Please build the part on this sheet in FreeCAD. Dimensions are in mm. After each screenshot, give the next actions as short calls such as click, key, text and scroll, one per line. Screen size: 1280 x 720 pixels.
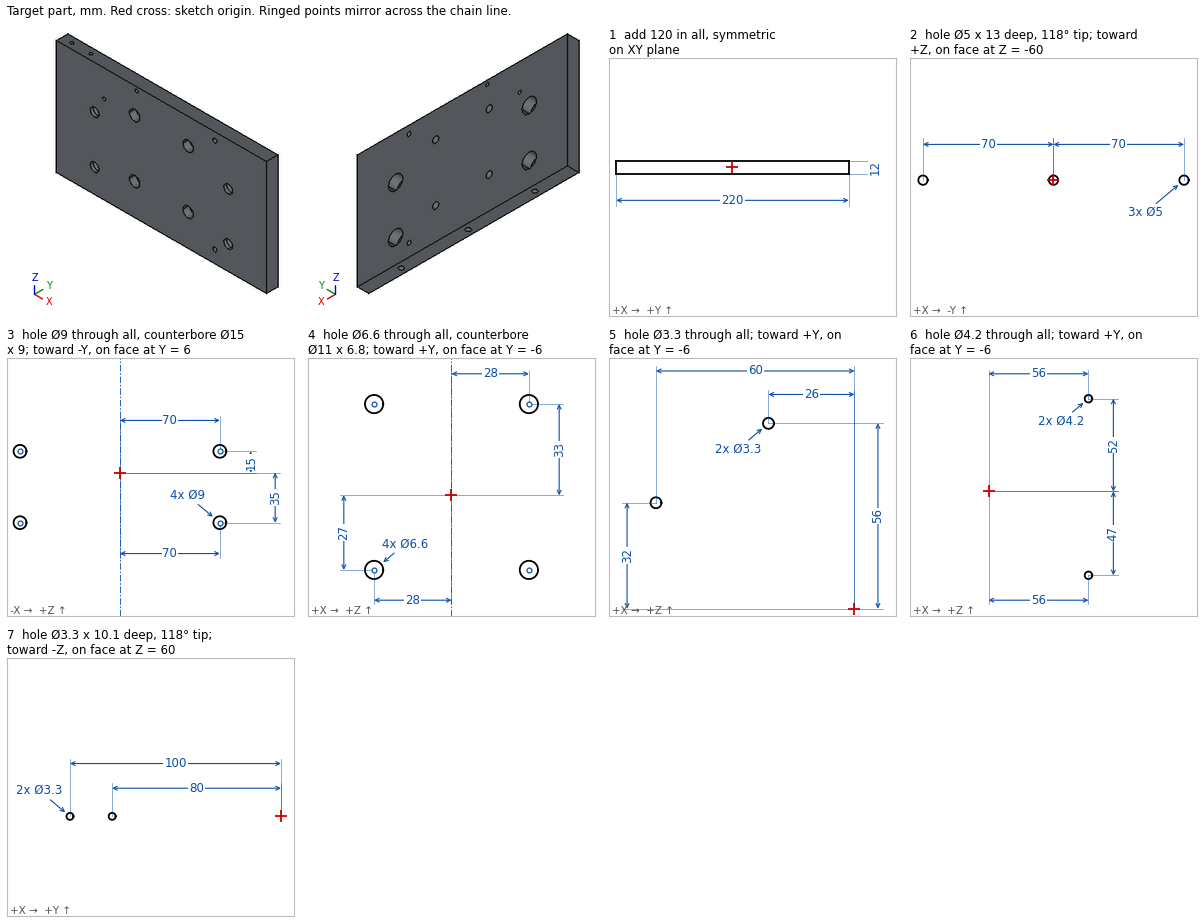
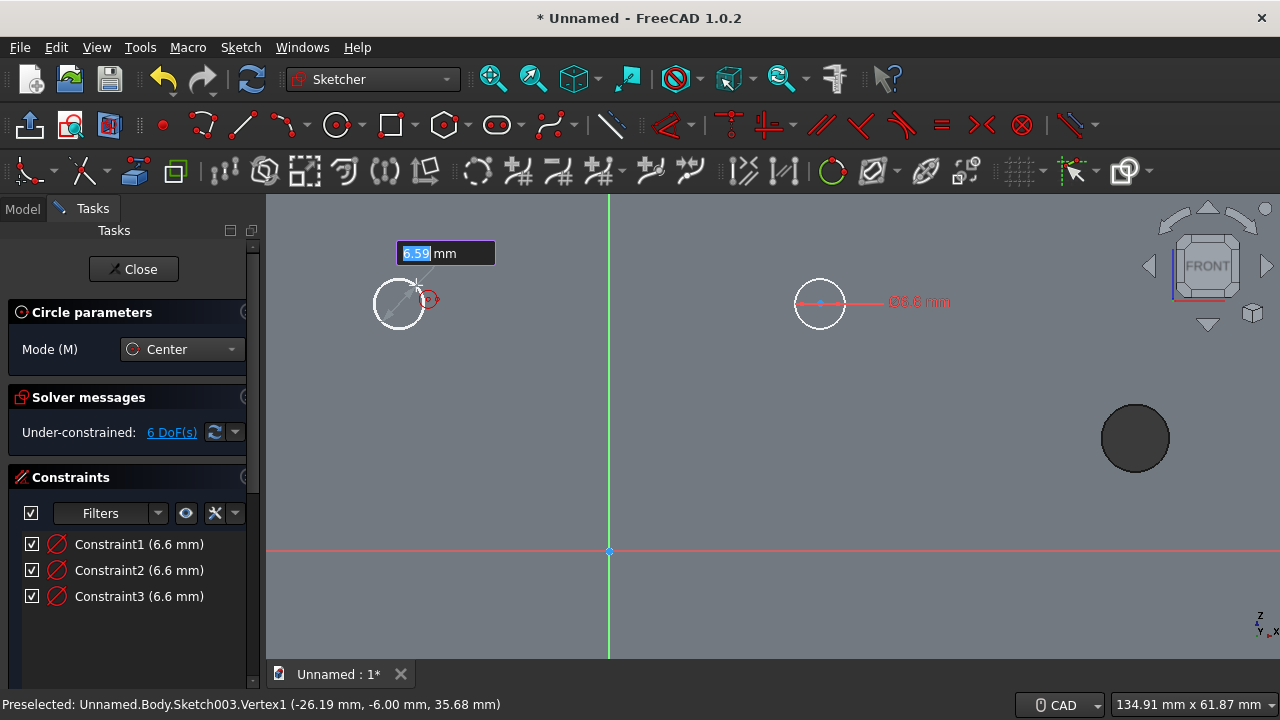
text(6.6)
key(Return)
key(Escape)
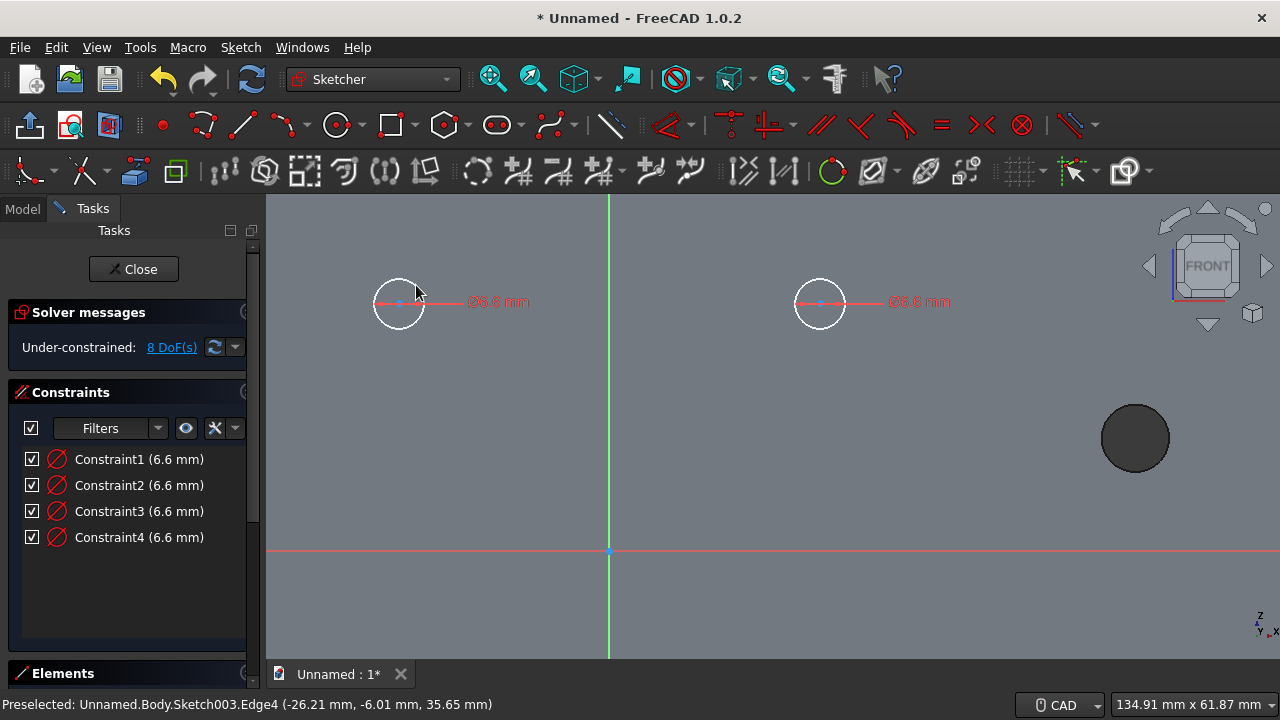
scroll(820, 302, down, 3)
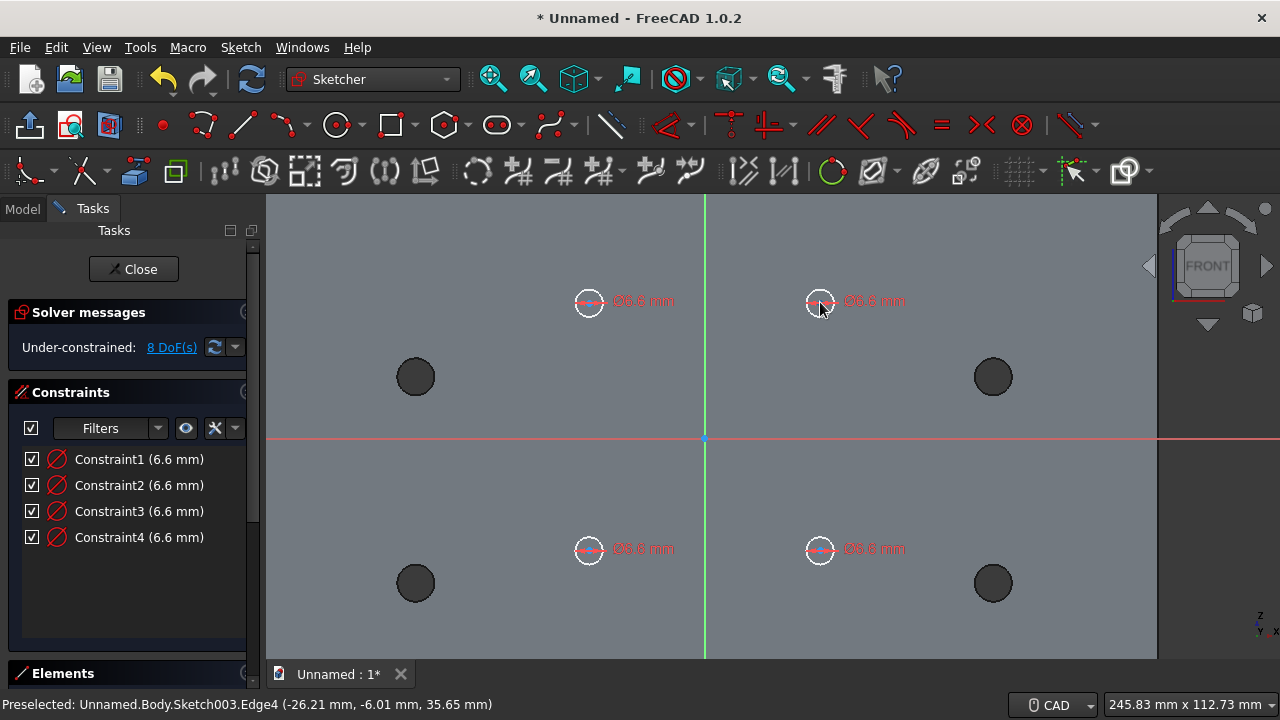
click(589, 551)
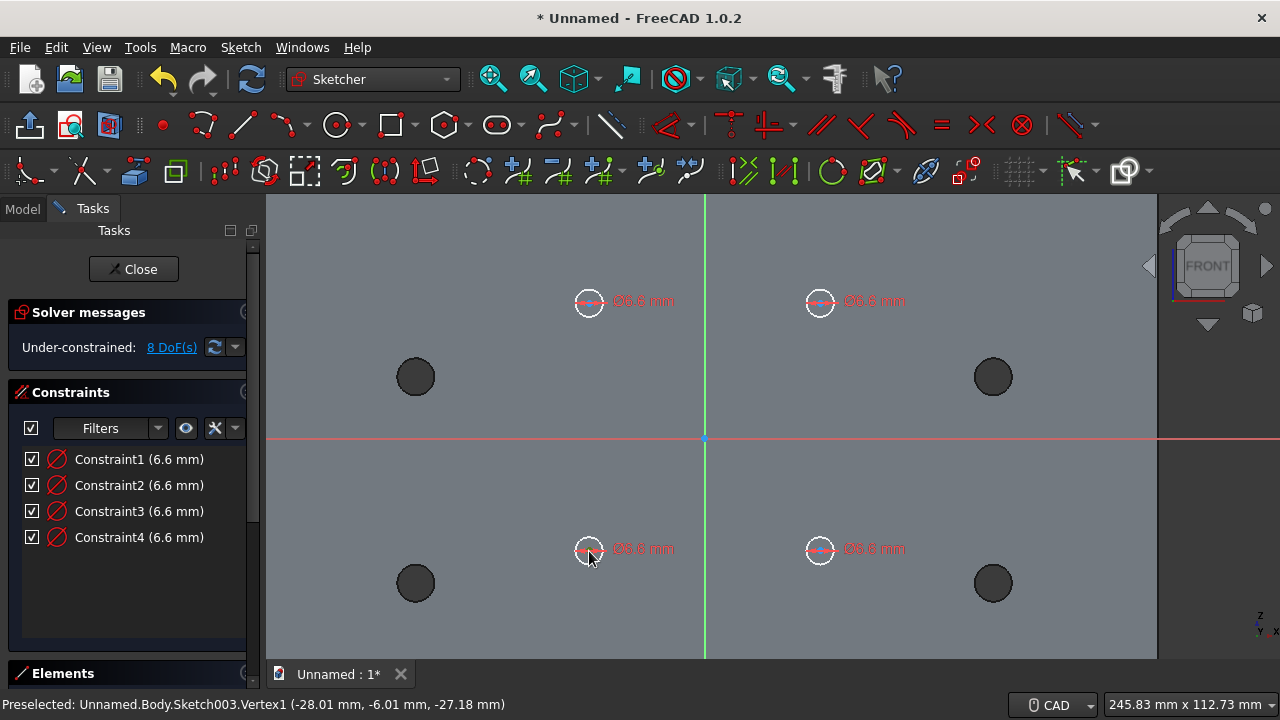
click(820, 551)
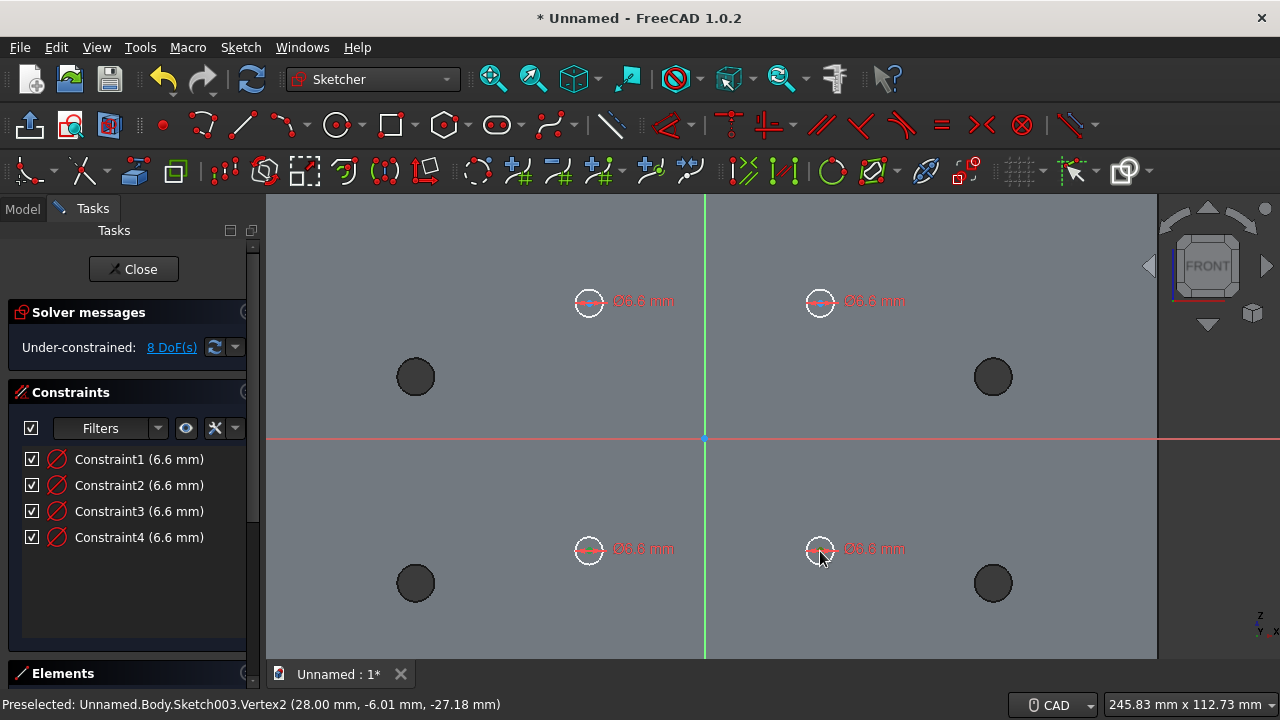
click(705, 602)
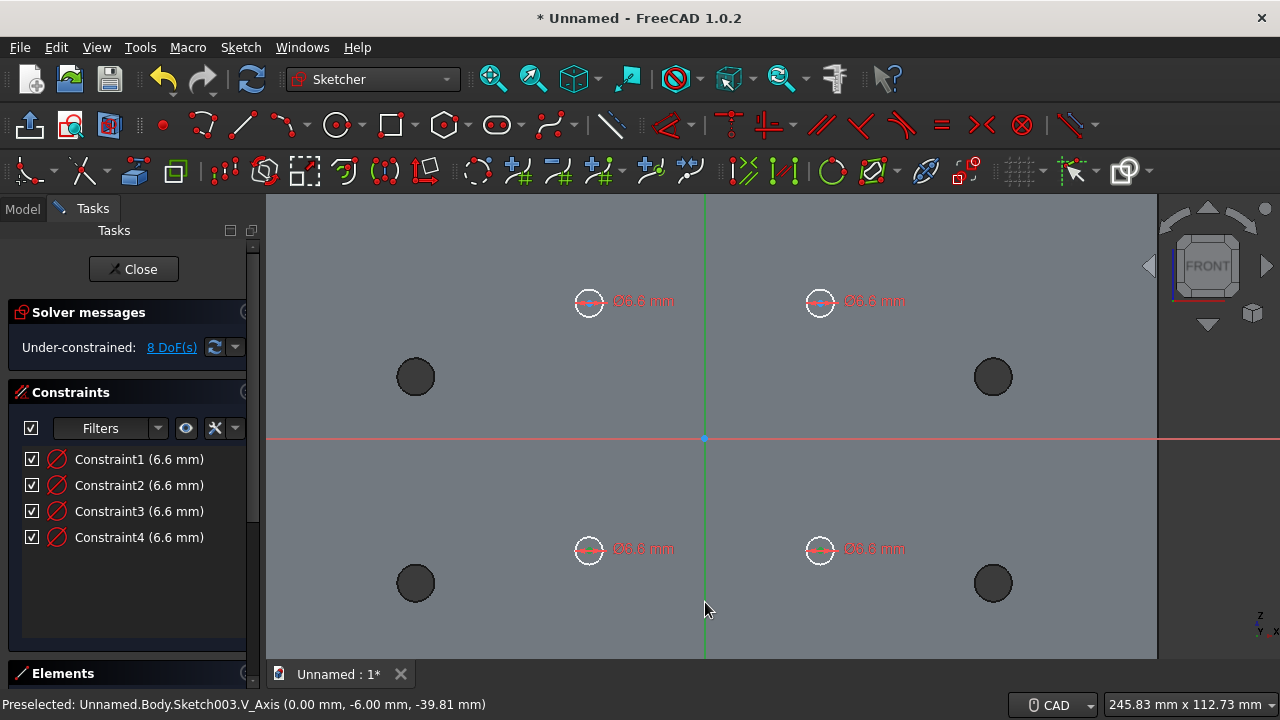
key(s)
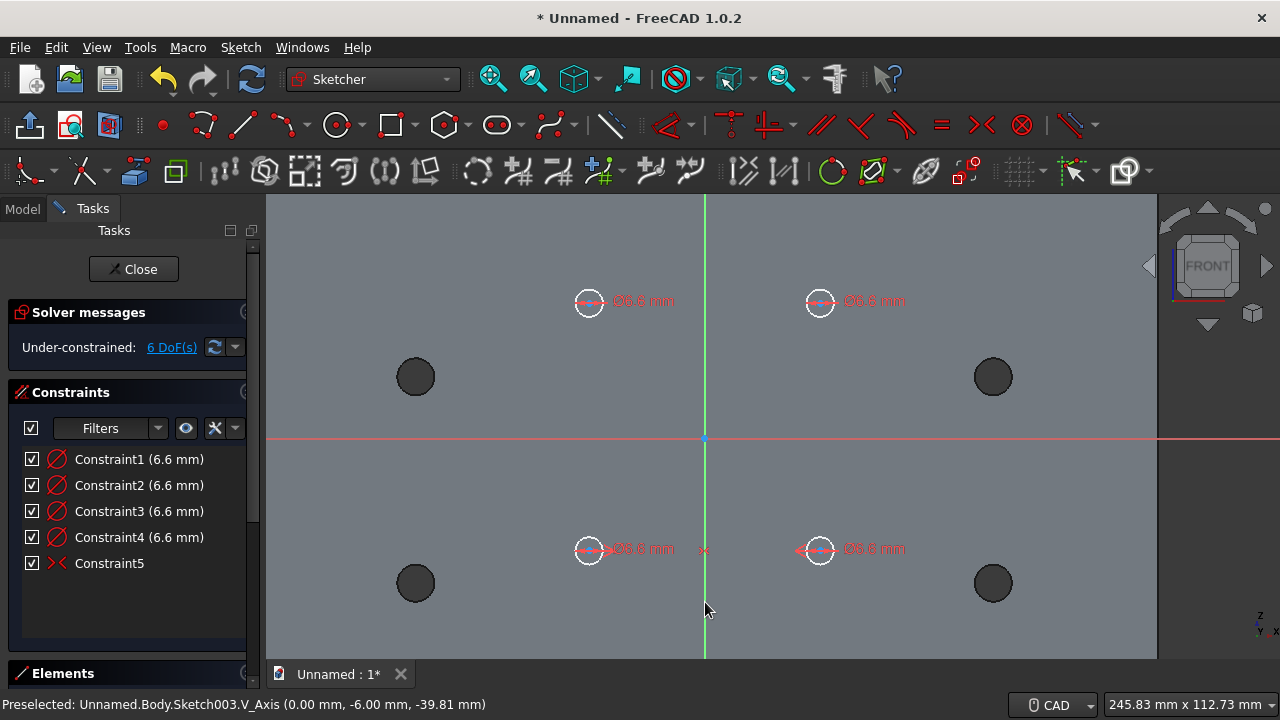
click(820, 303)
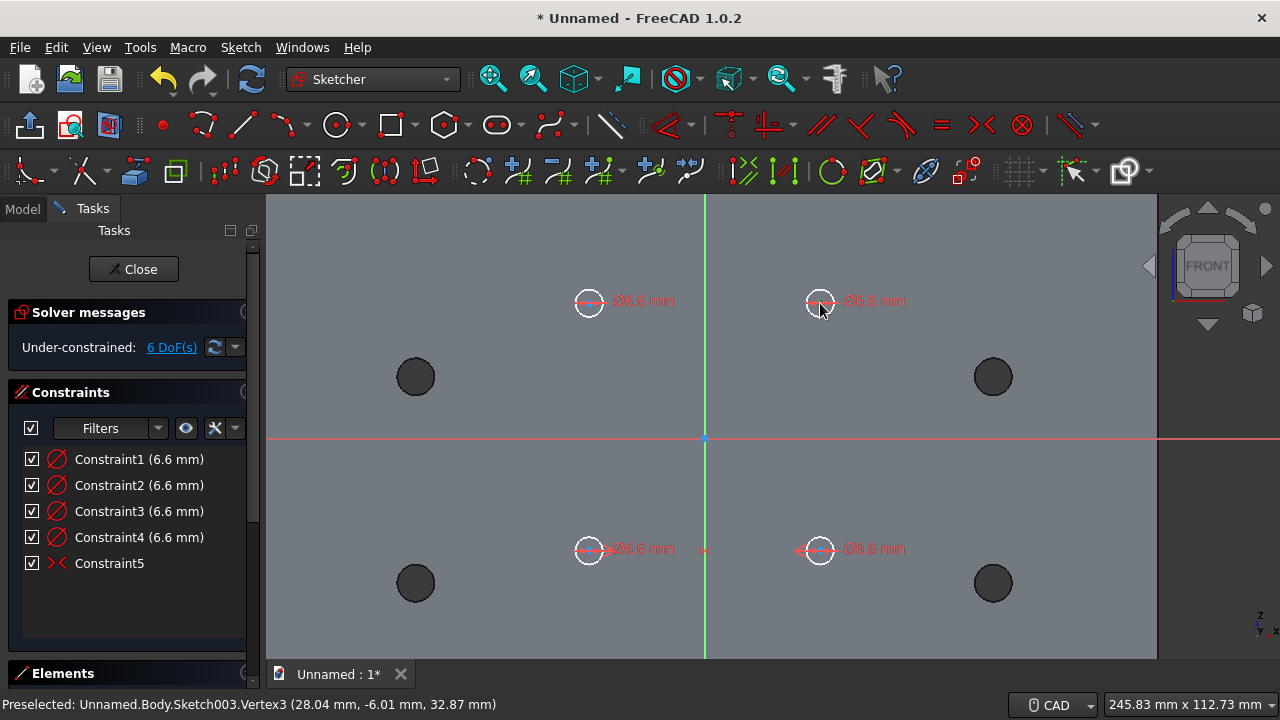
click(589, 303)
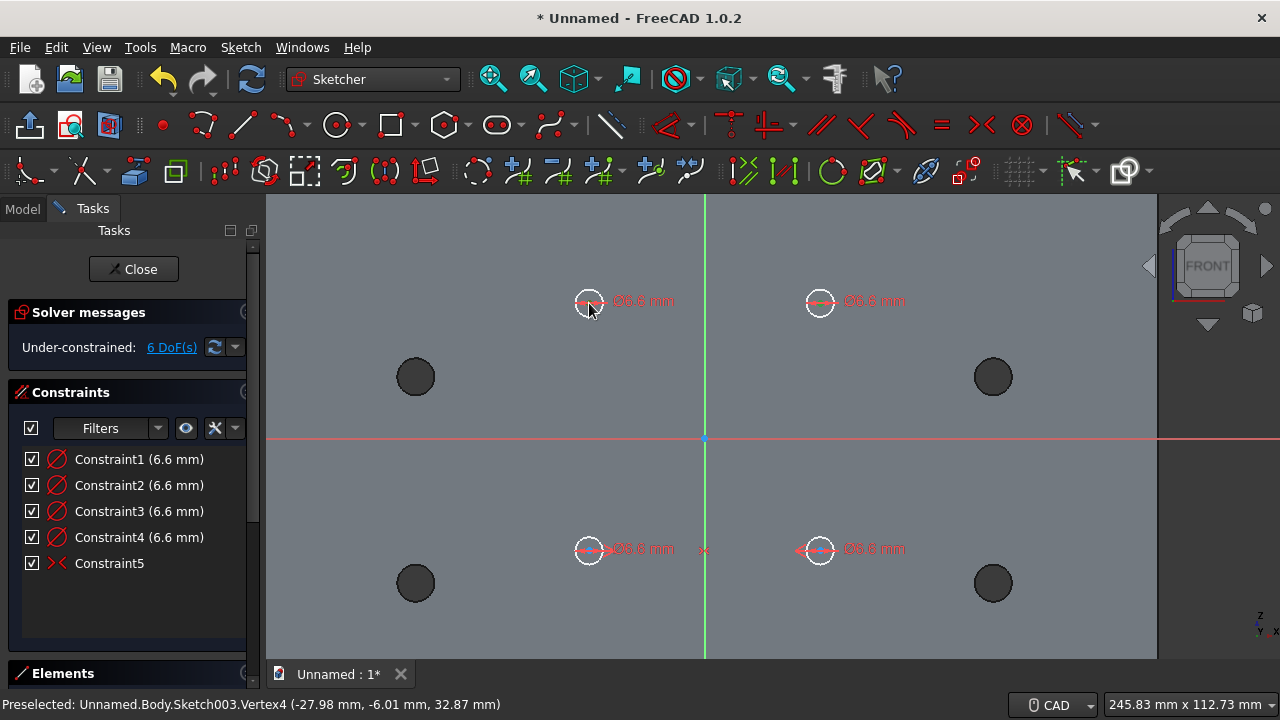
click(705, 602)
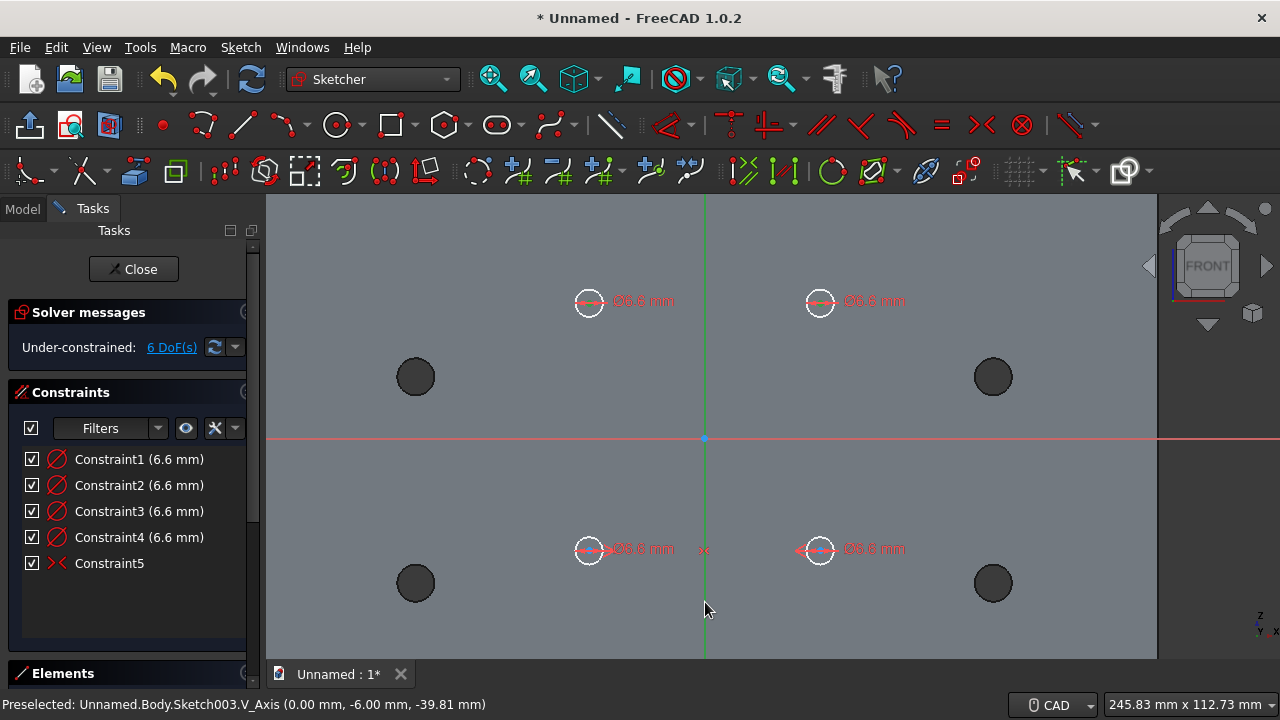
click(982, 126)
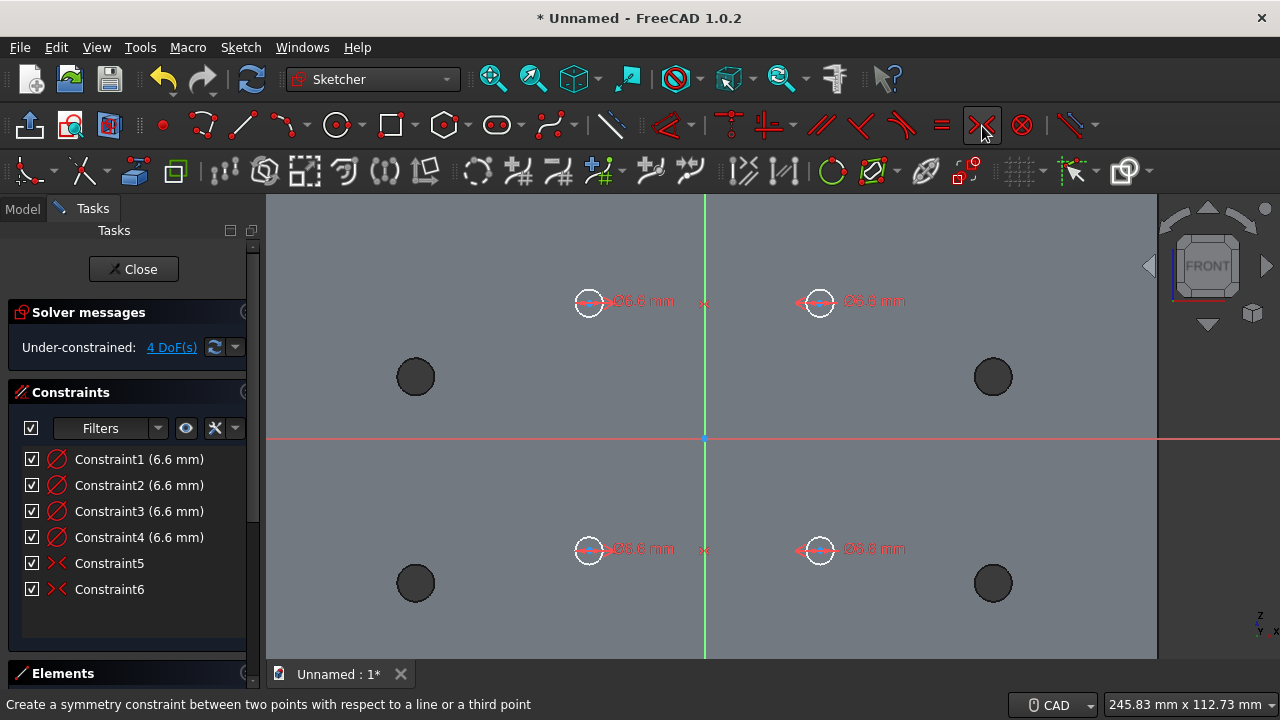
click(666, 126)